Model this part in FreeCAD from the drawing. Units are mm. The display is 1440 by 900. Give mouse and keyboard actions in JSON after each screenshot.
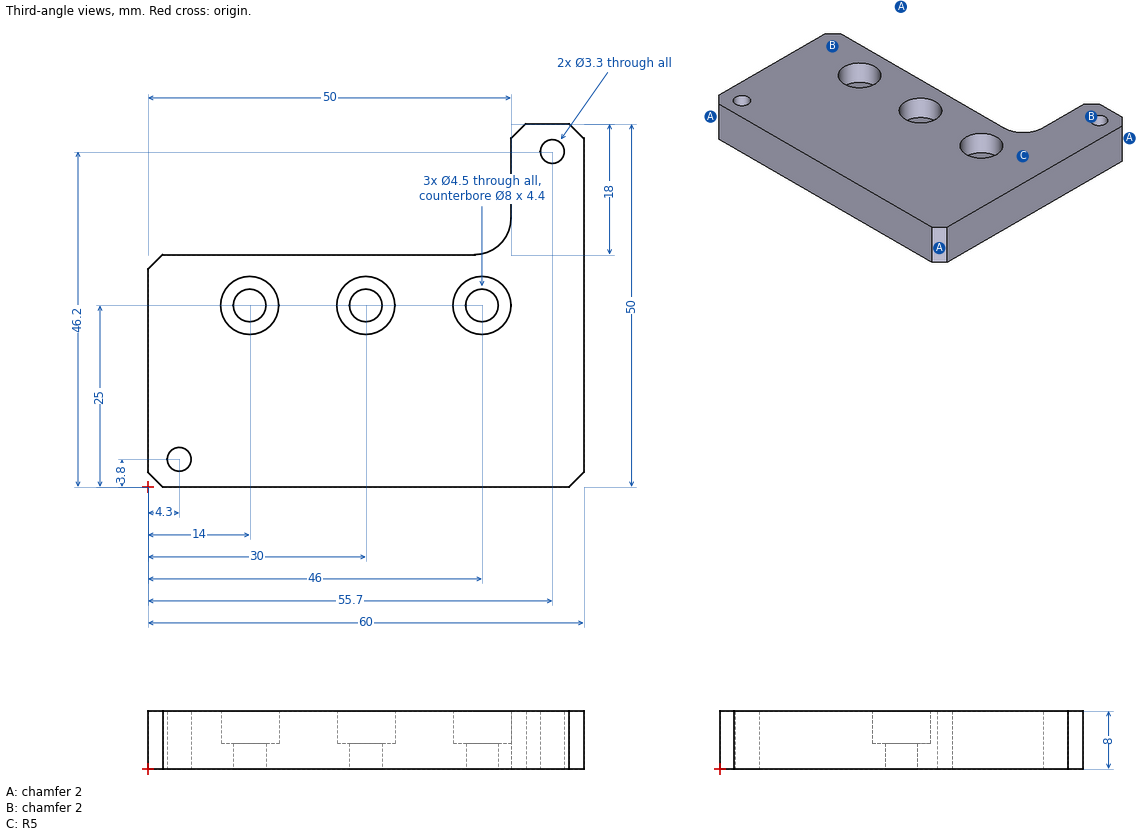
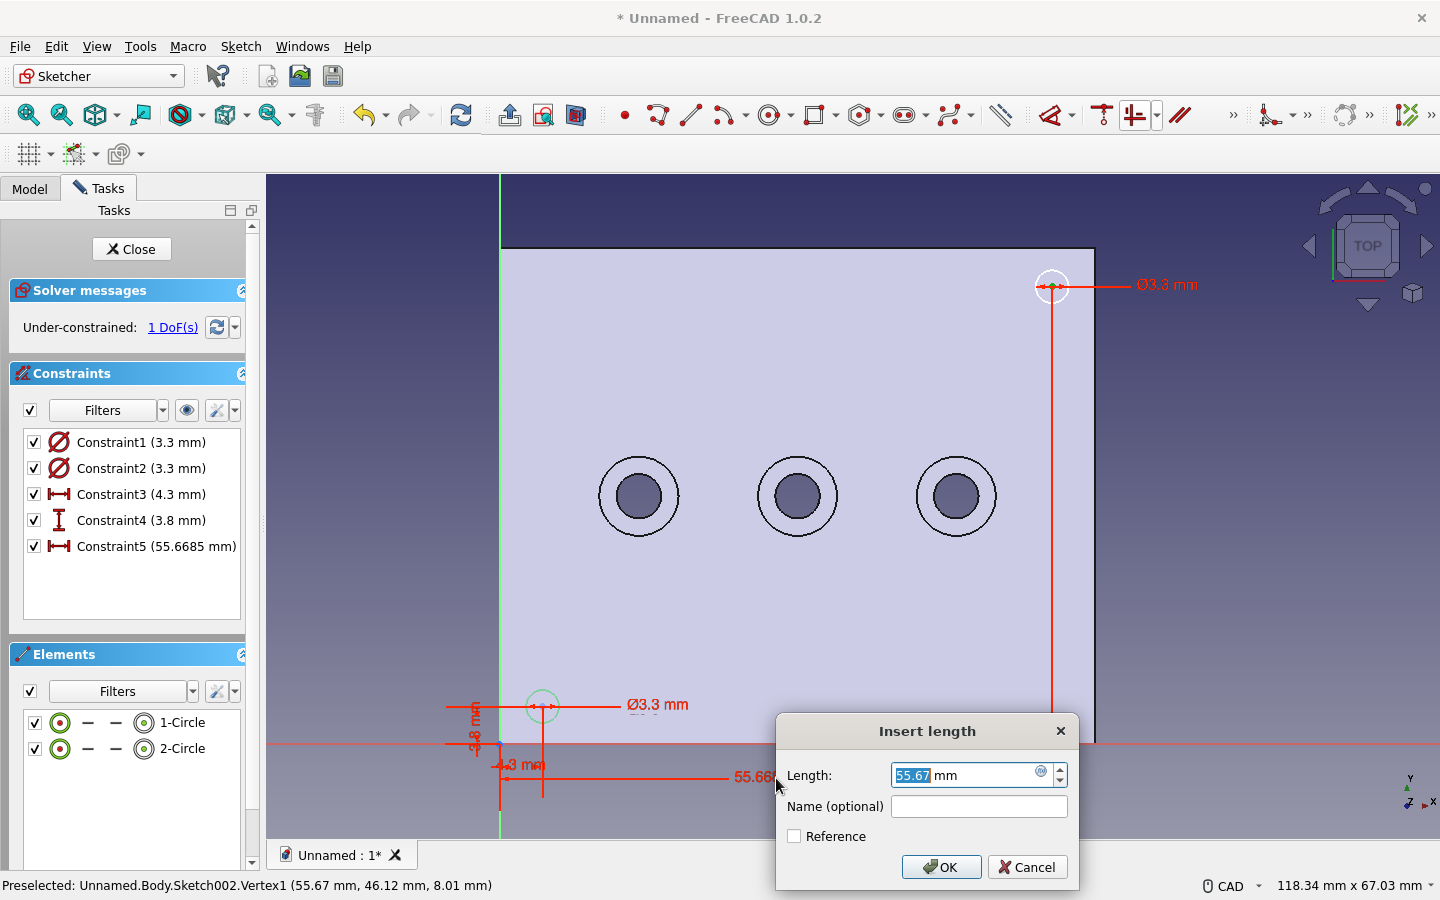
{"action": "type", "text": "55.7"}
{"action": "key", "text": "Return"}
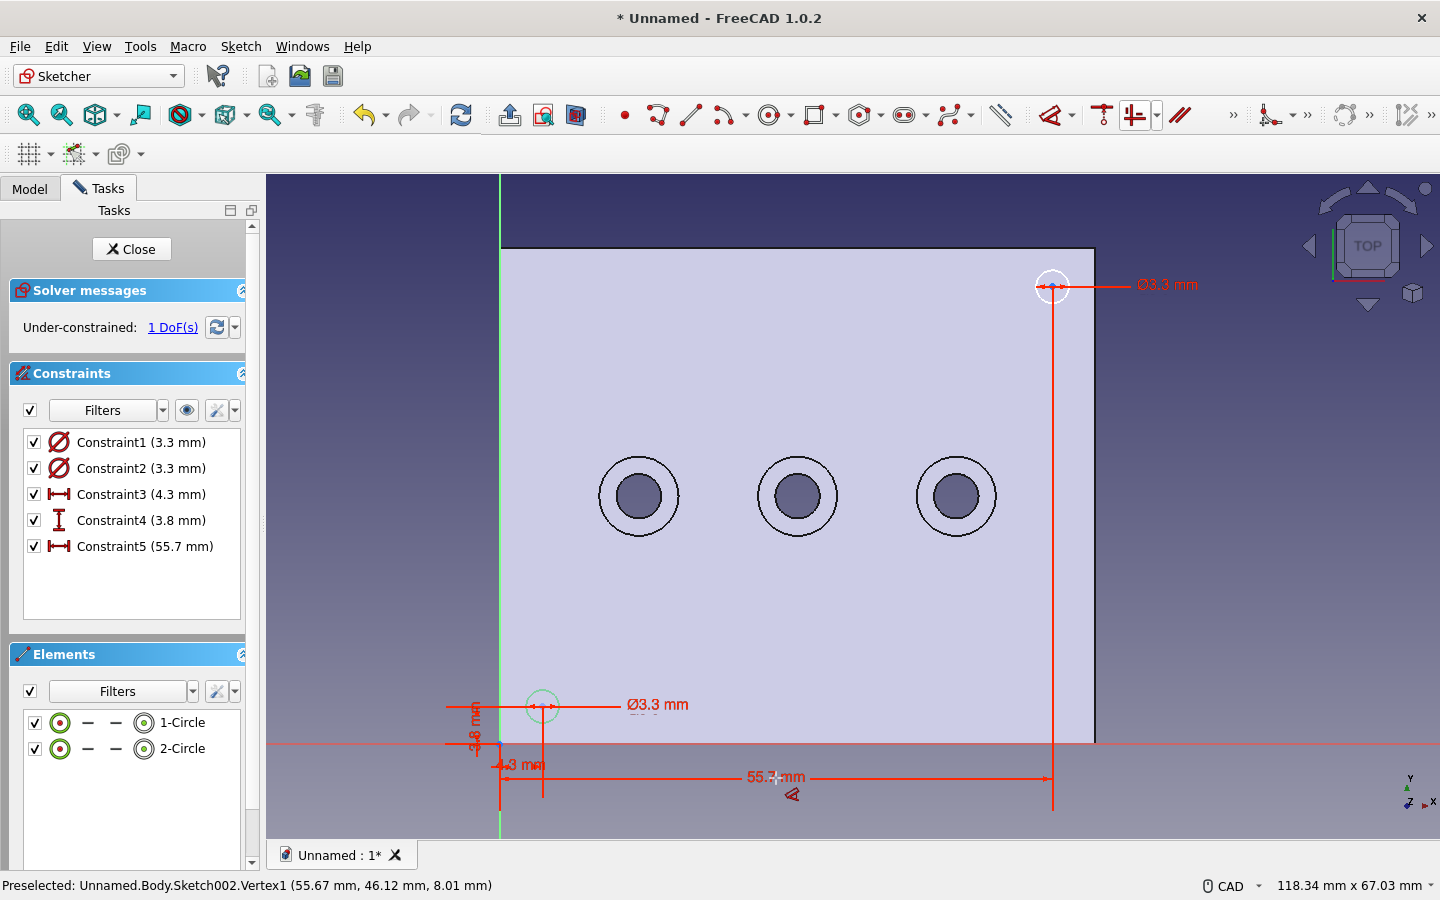
{"action": "left_click", "coordinate": [1053, 287]}
{"action": "left_click", "coordinate": [466, 515]}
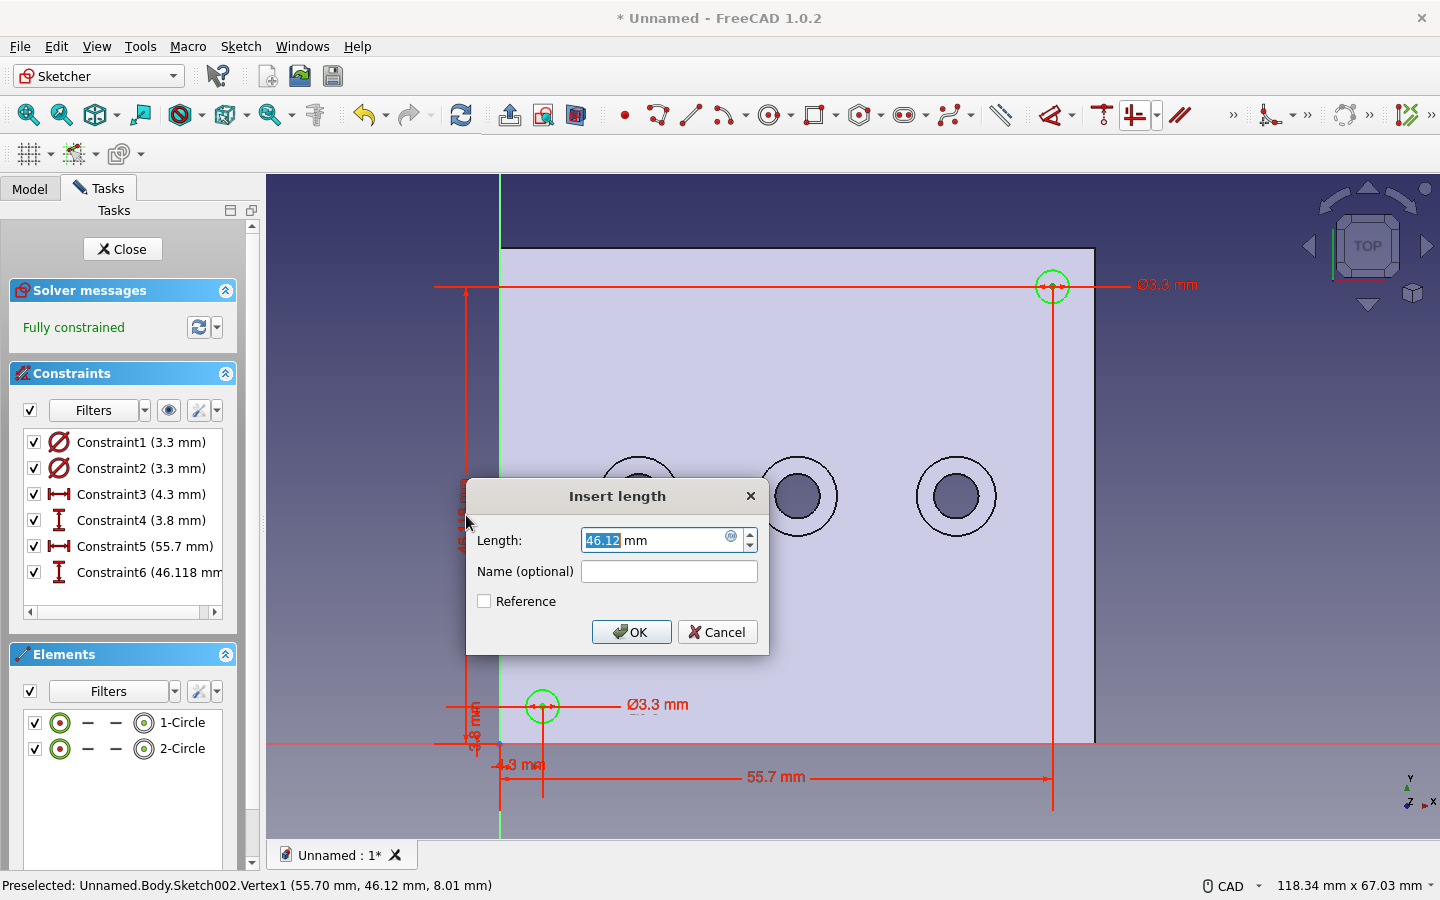
{"action": "type", "text": "46.2"}
{"action": "key", "text": "Return"}
{"action": "key", "text": "Escape"}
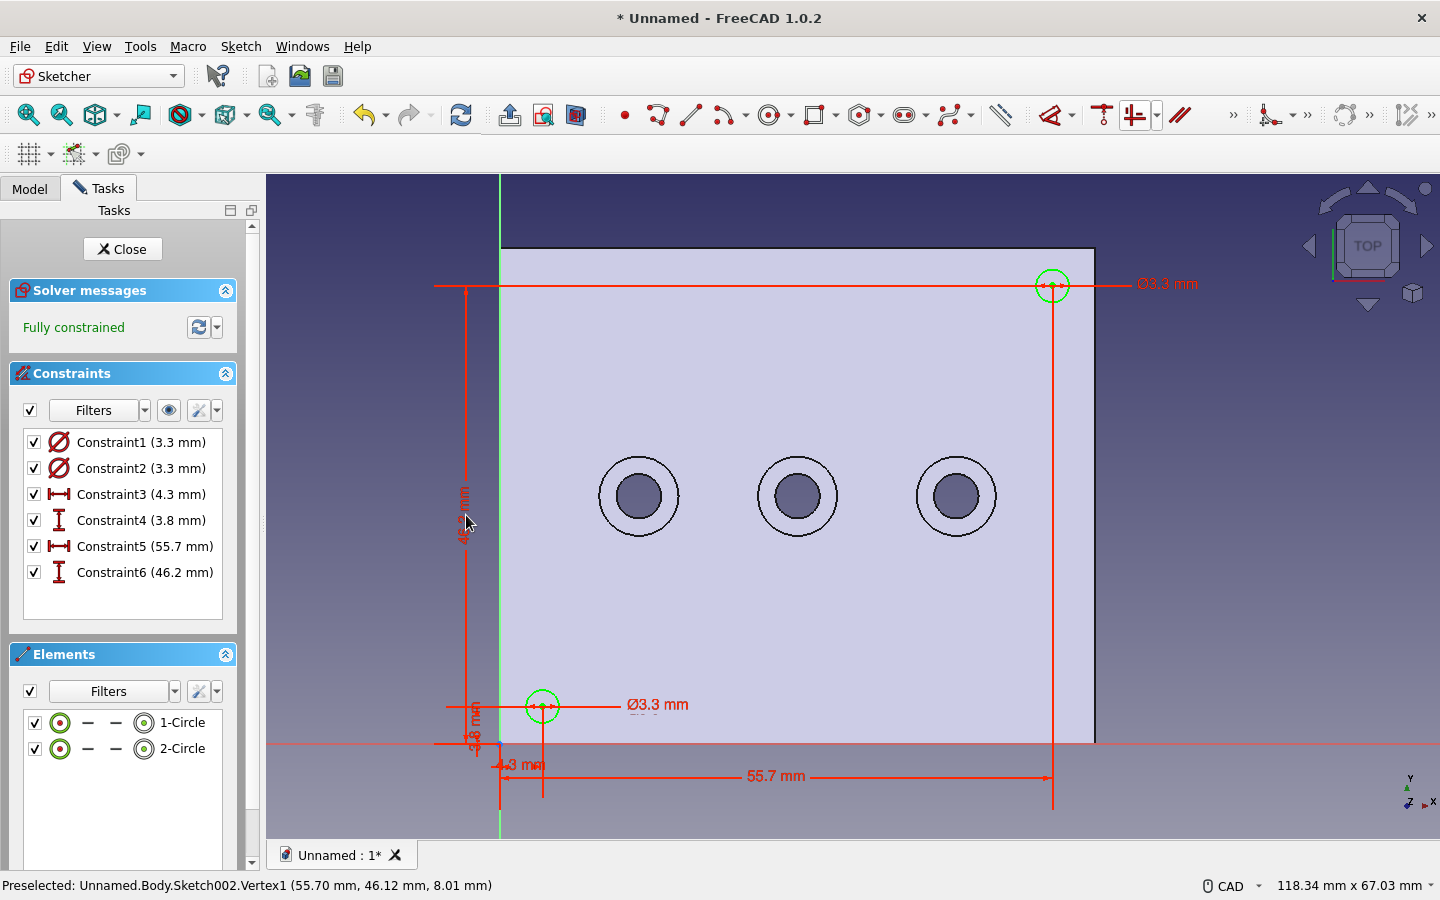
{"action": "left_click", "coordinate": [123, 249]}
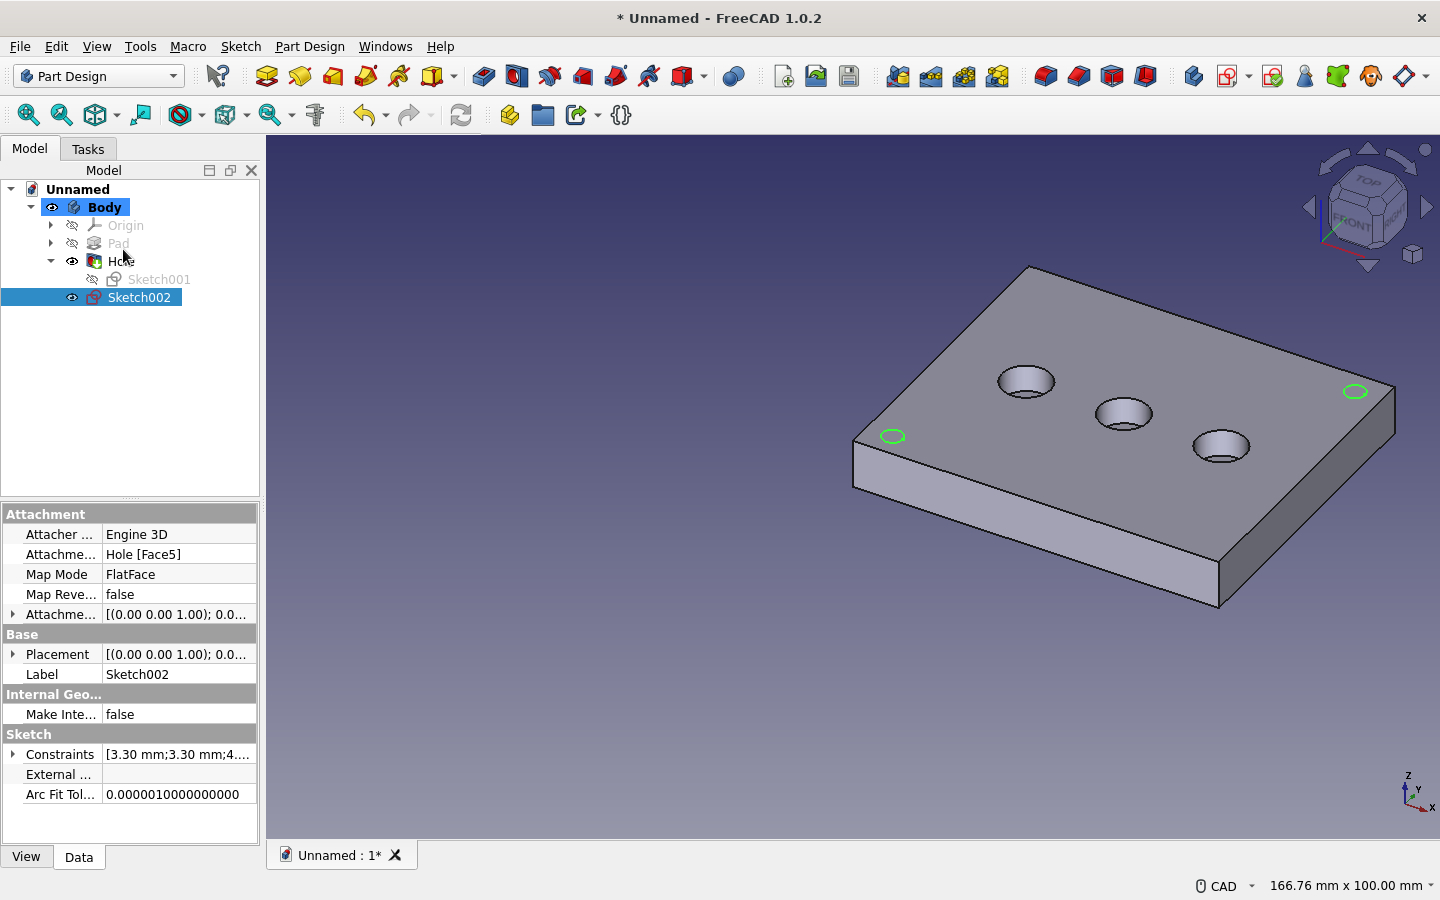
{"action": "left_click", "coordinate": [517, 76]}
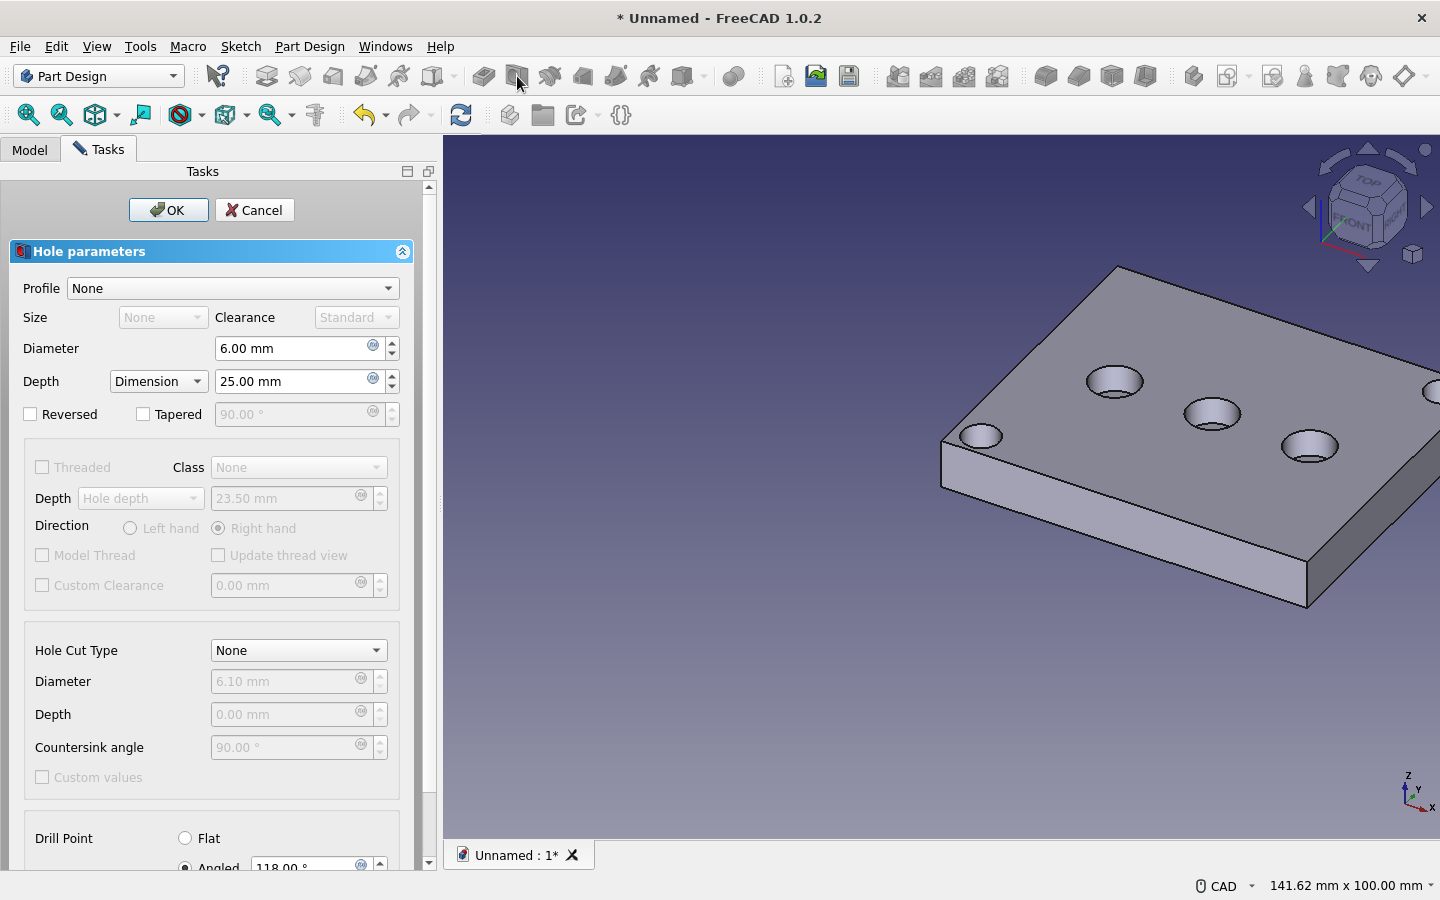
{"action": "triple_click", "coordinate": [300, 348]}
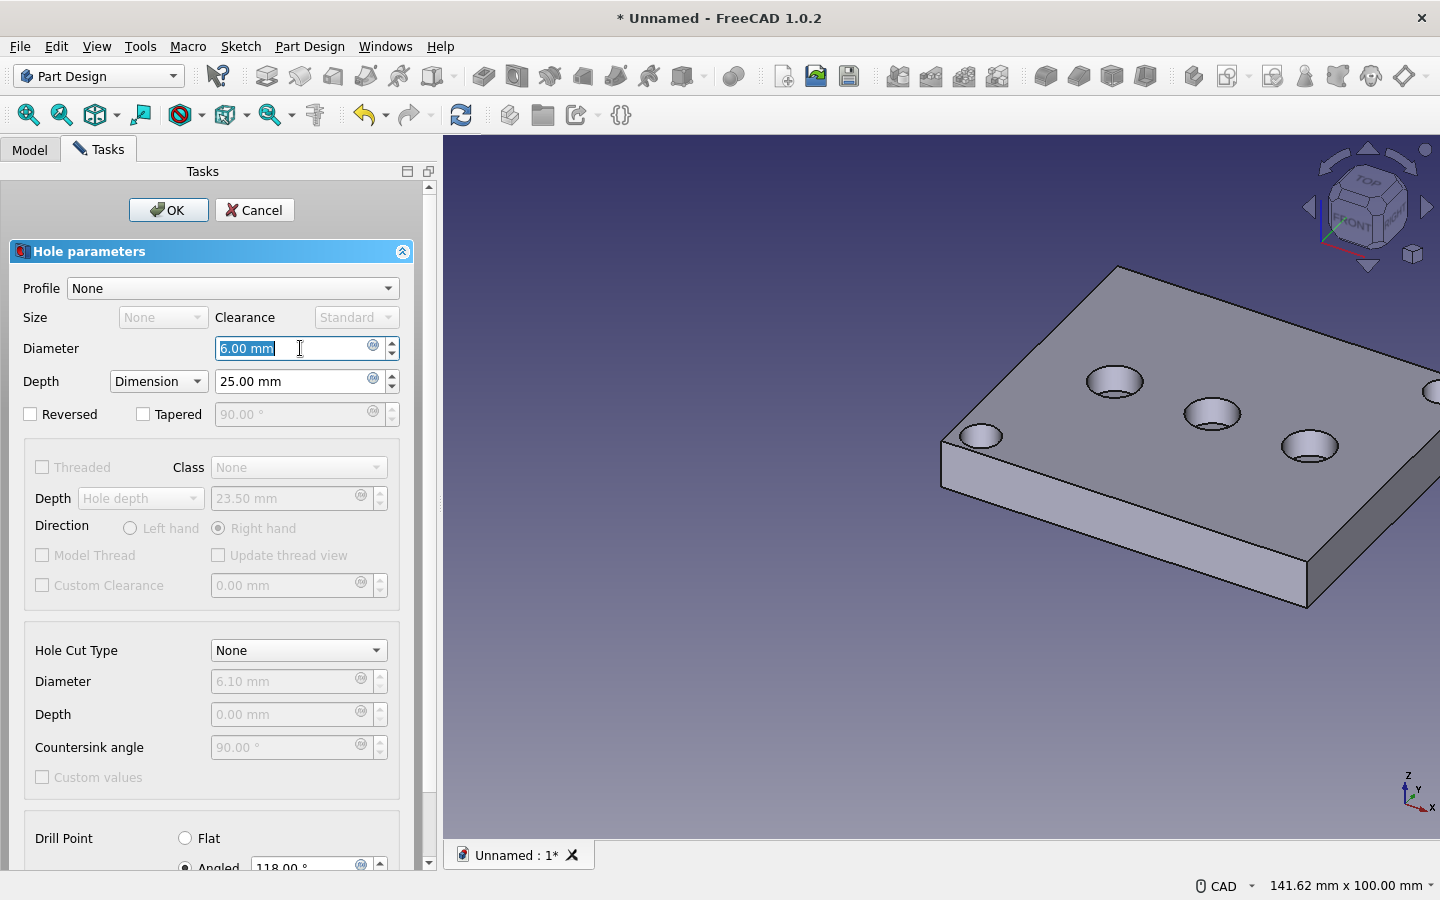
{"action": "type", "text": "3.3"}
{"action": "key", "text": "Tab"}